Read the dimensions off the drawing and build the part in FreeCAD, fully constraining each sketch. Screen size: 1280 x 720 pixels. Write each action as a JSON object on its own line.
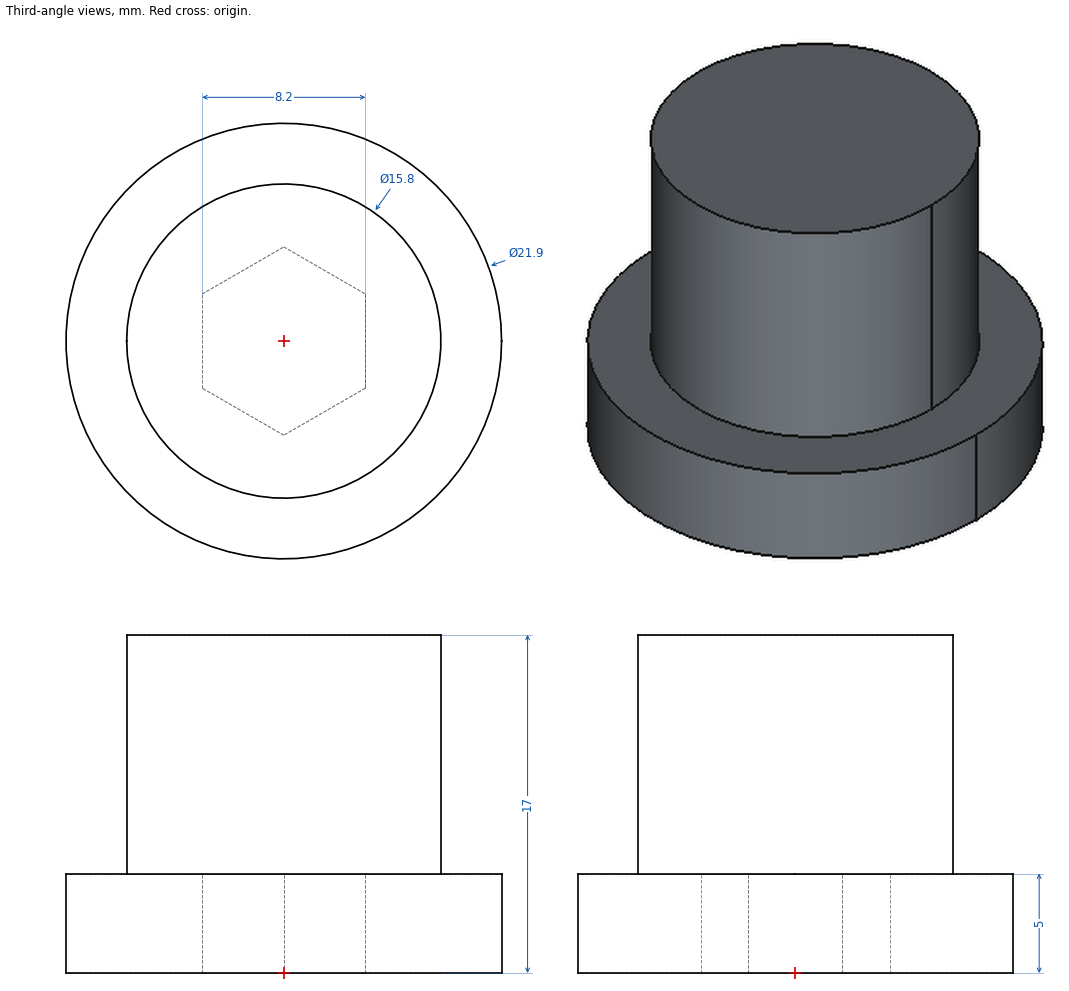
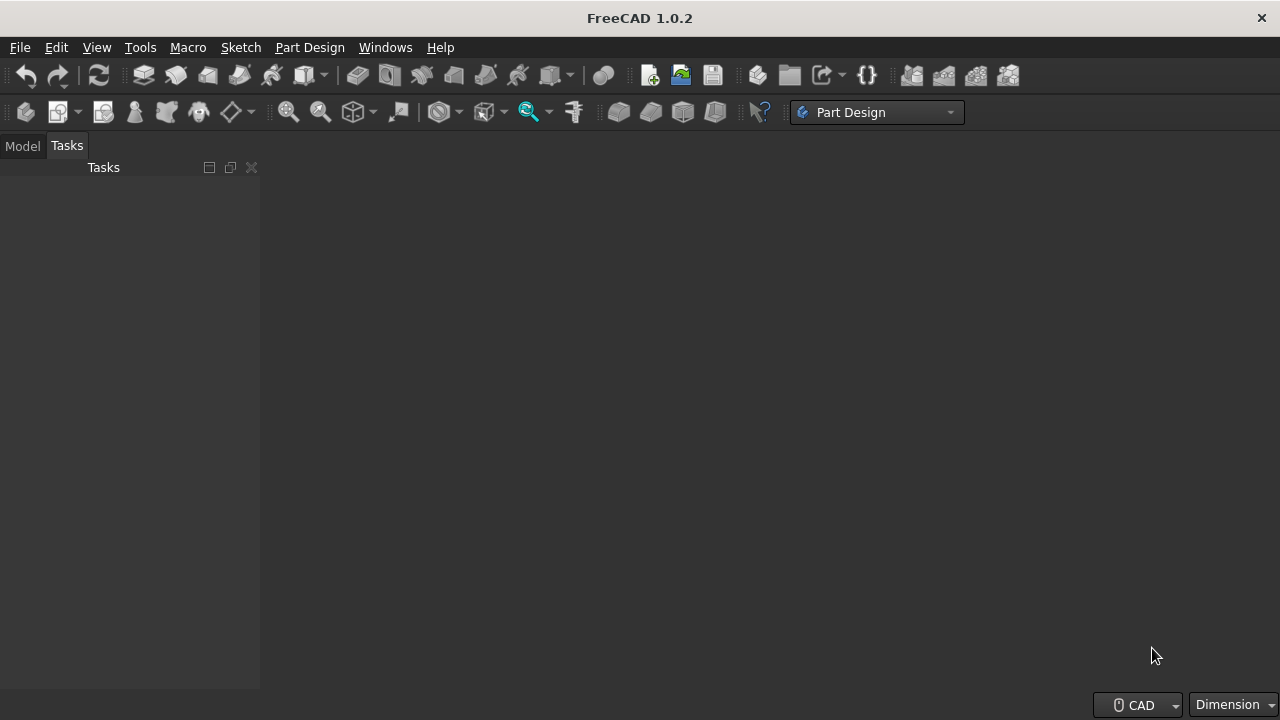
{"action": "left_click", "coordinate": [650, 76]}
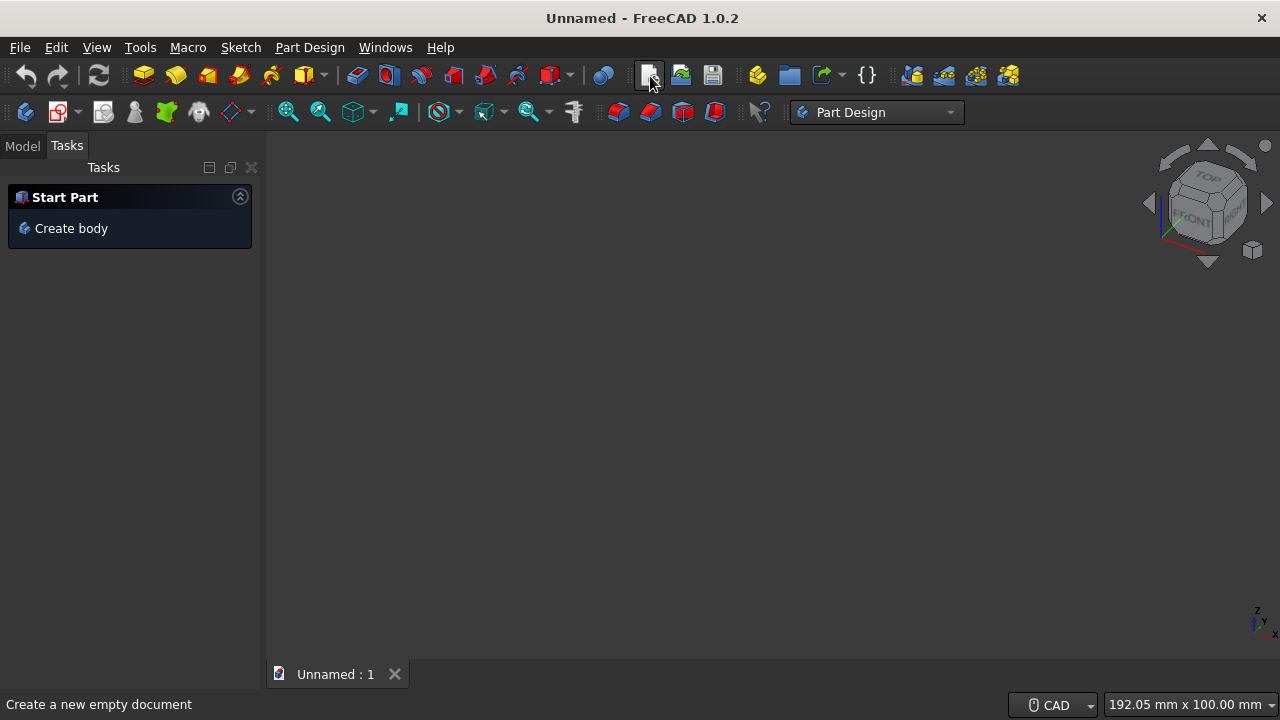
{"action": "left_click", "coordinate": [58, 112]}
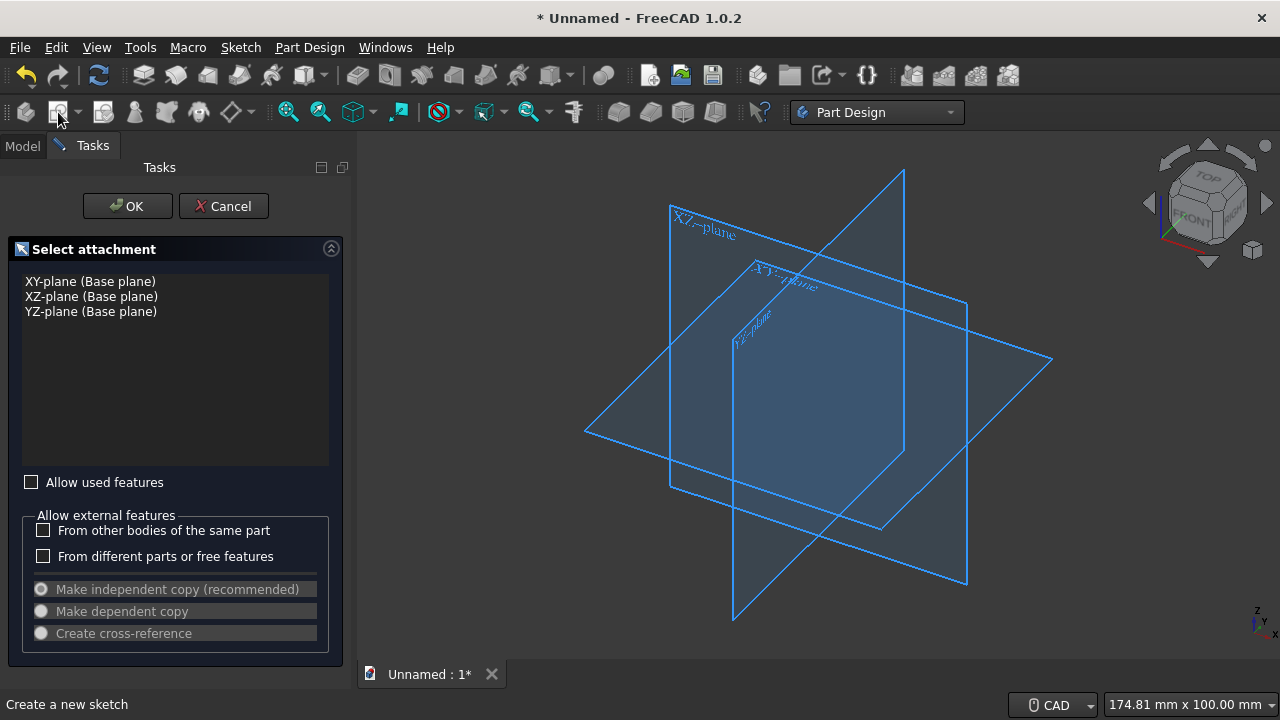
{"action": "left_click", "coordinate": [82, 282]}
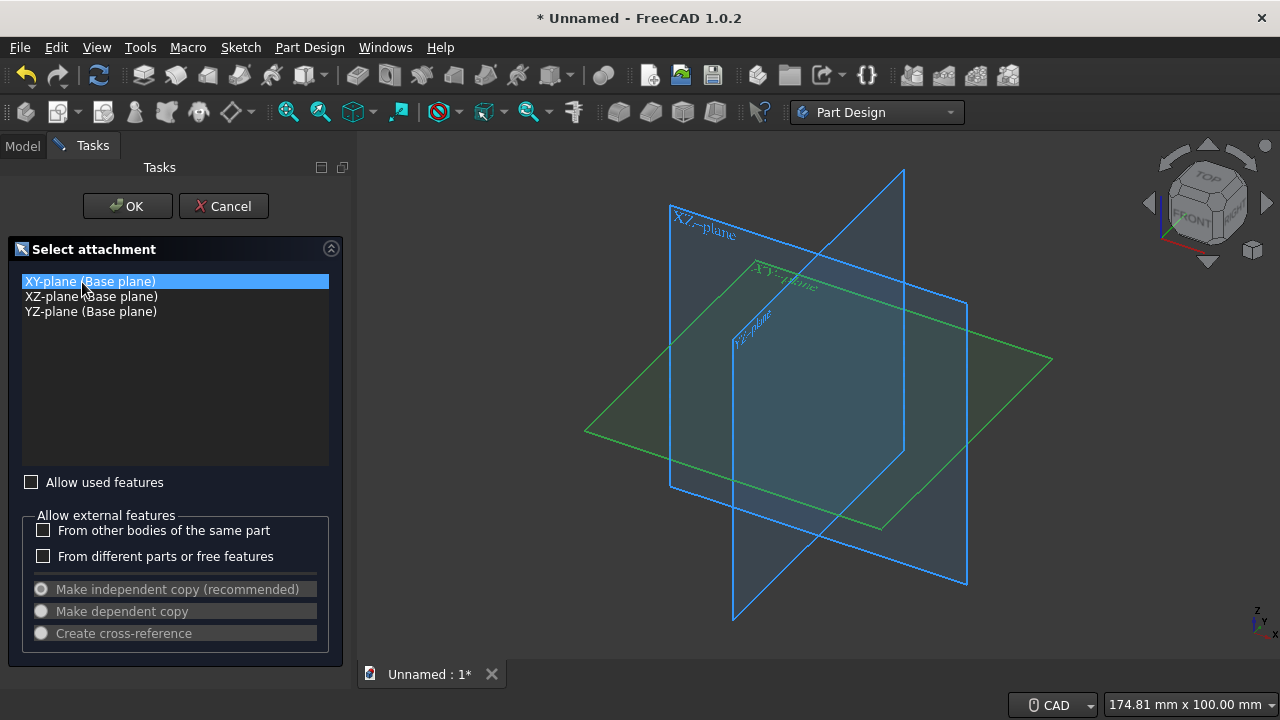
{"action": "left_click", "coordinate": [128, 206]}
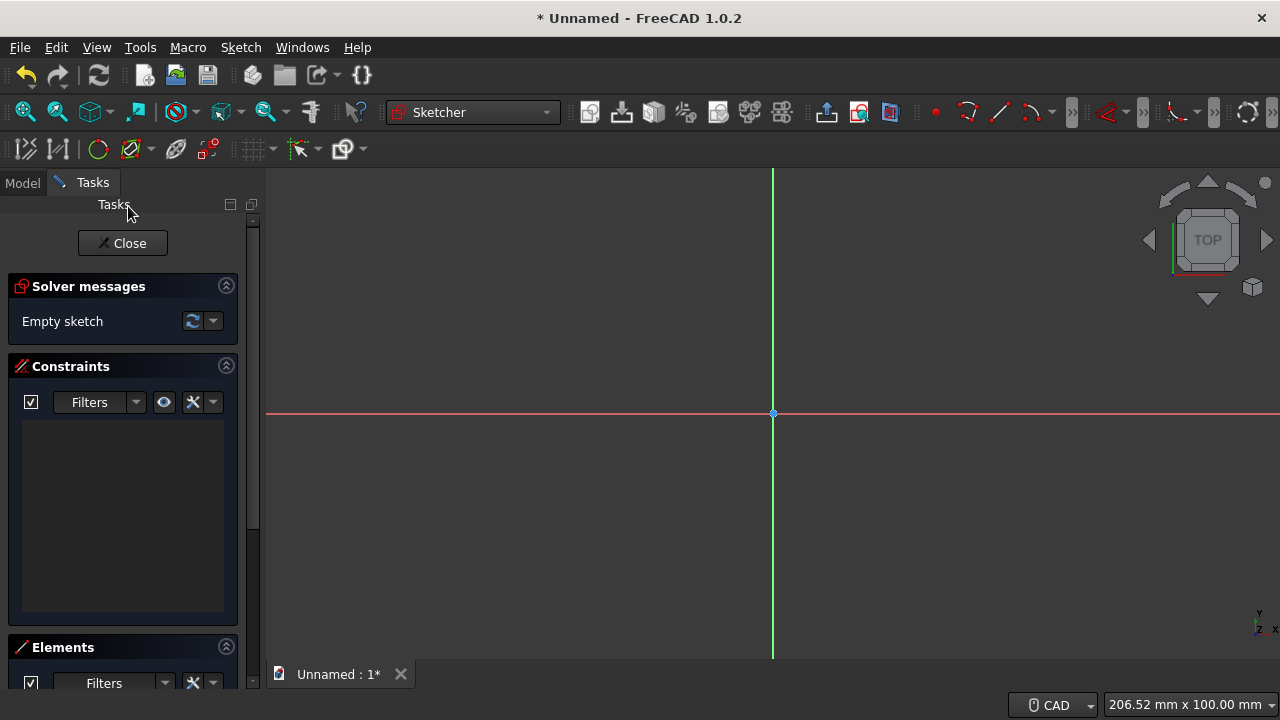
{"action": "scroll", "coordinate": [813, 414], "scroll_direction": "up", "scroll_amount": 5}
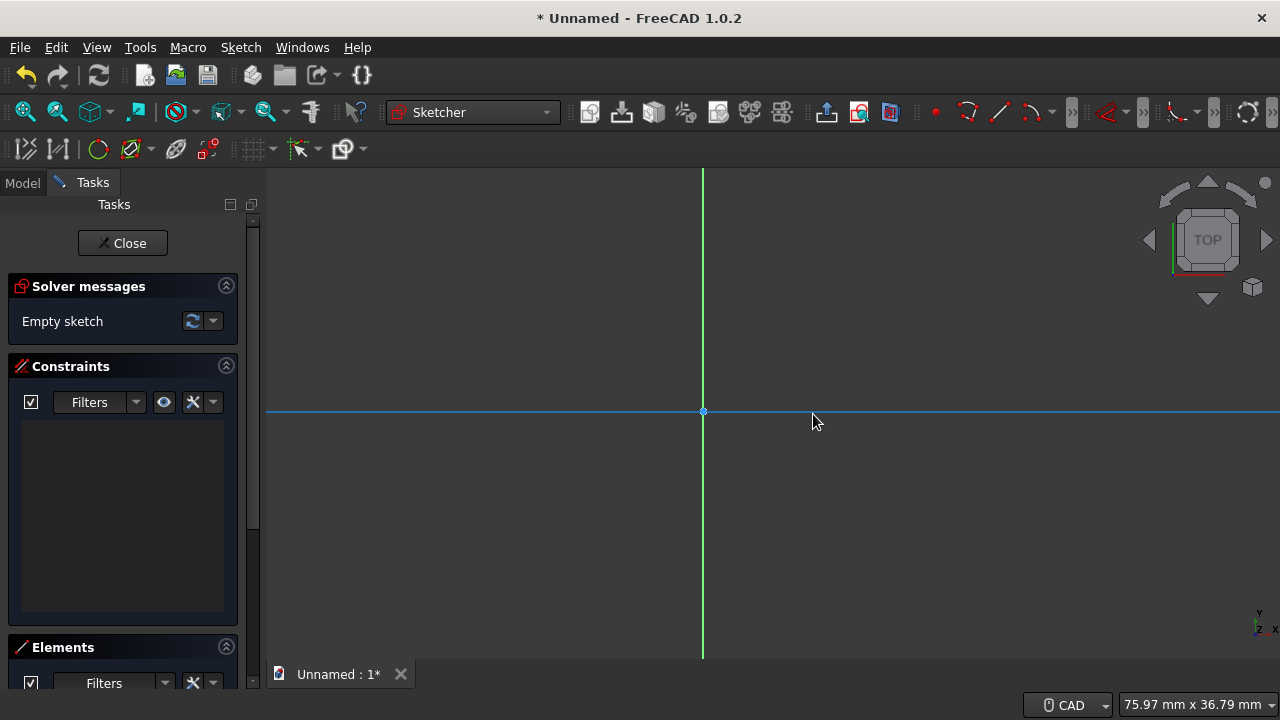
{"action": "key", "text": "g c"}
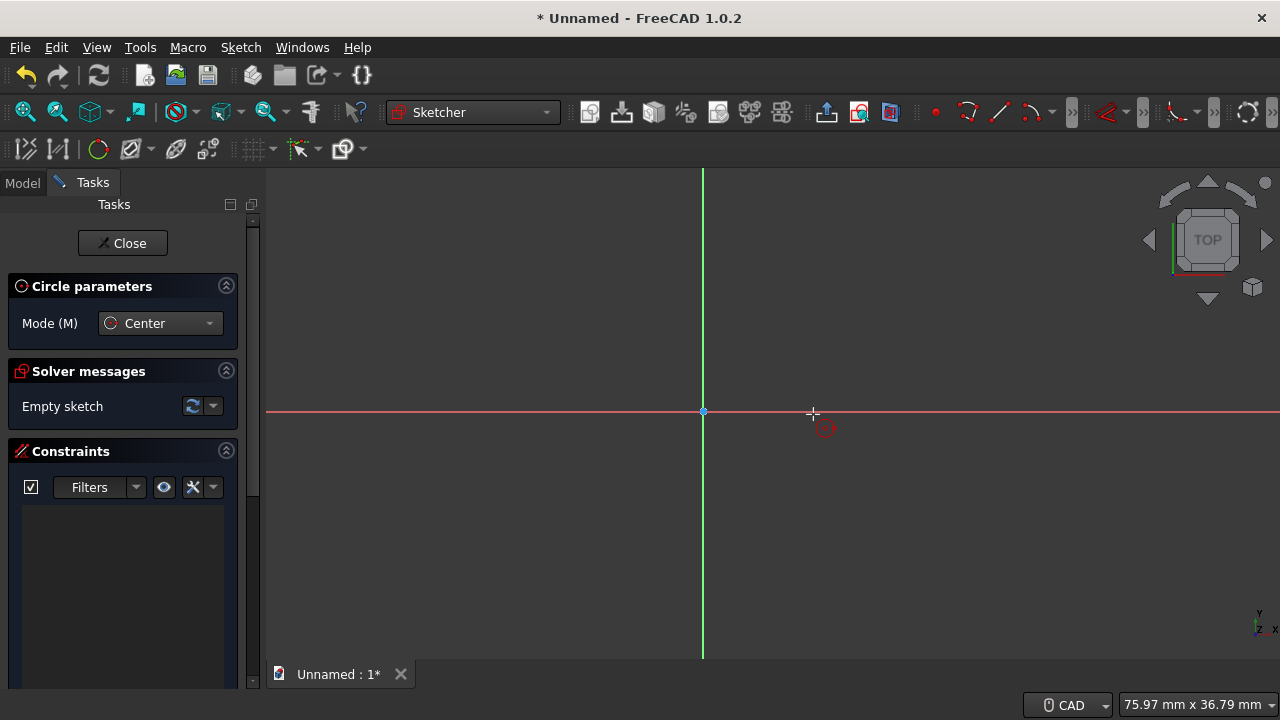
{"action": "left_click", "coordinate": [703, 412]}
{"action": "mouse_move", "coordinate": [807, 308]}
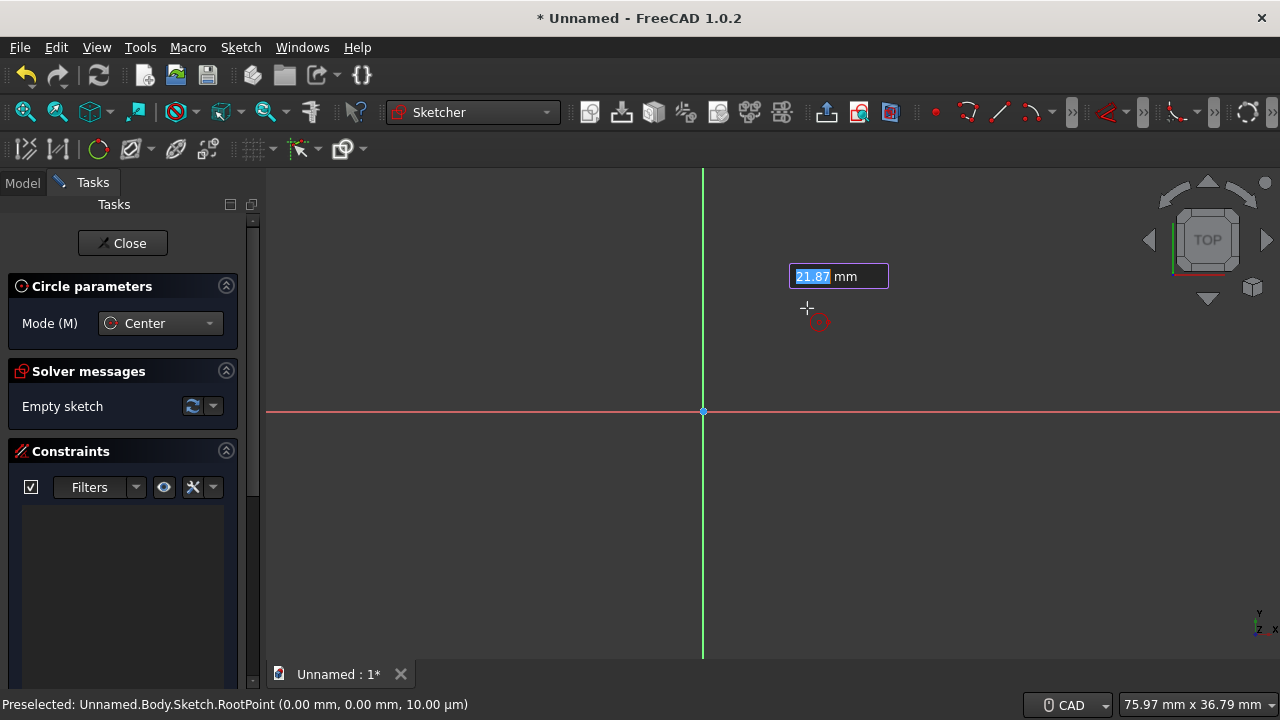
{"action": "type", "text": "21.9"}
{"action": "key", "text": "Return"}
{"action": "key", "text": "Escape"}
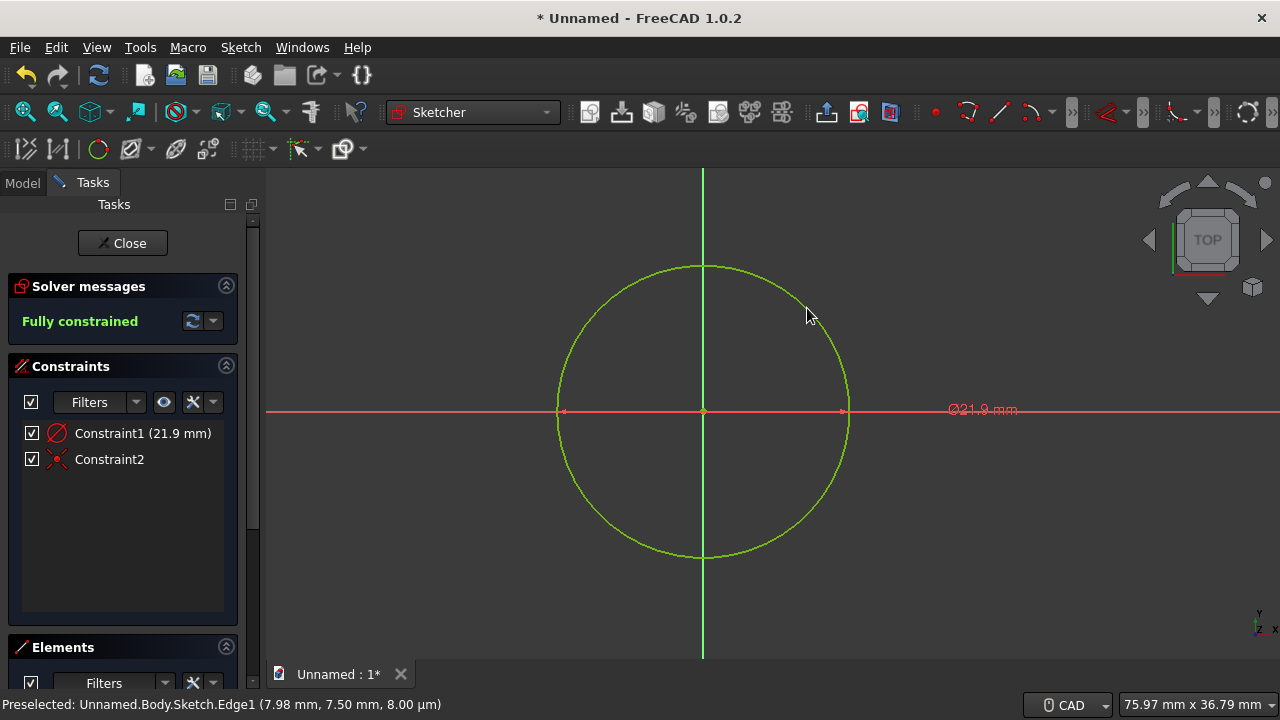
{"action": "left_click", "coordinate": [123, 243]}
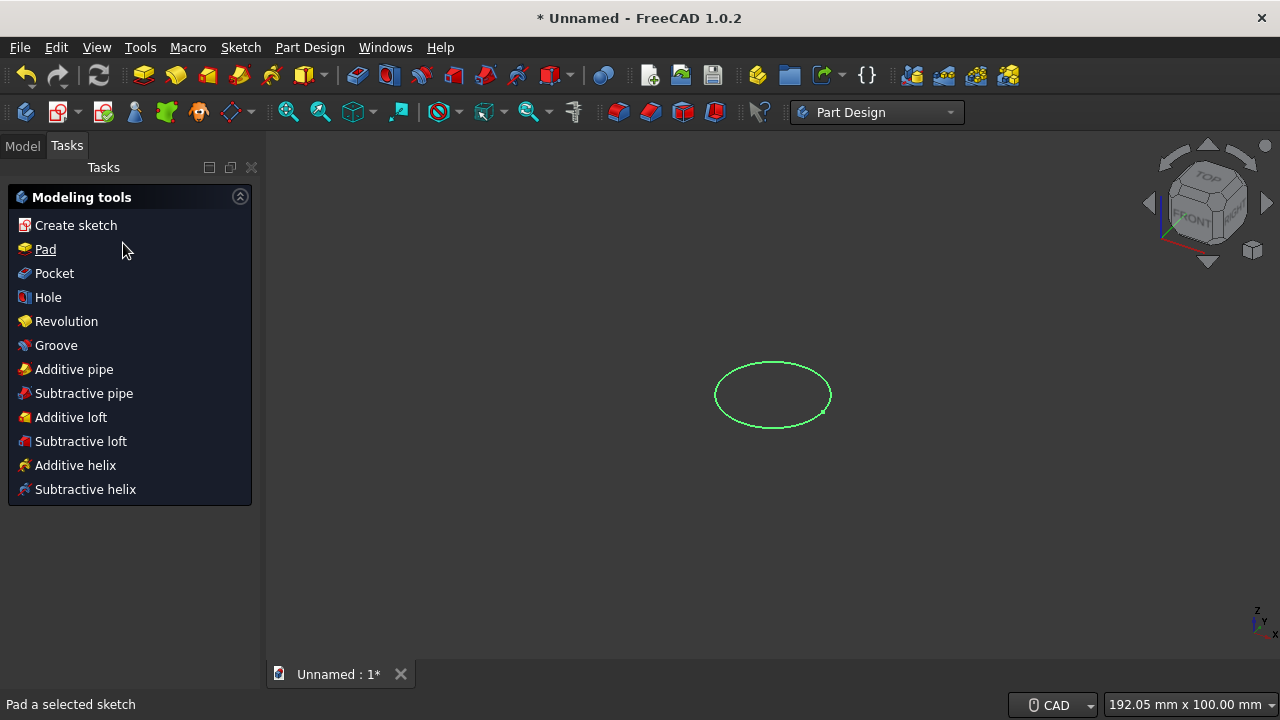
{"action": "left_click", "coordinate": [144, 76]}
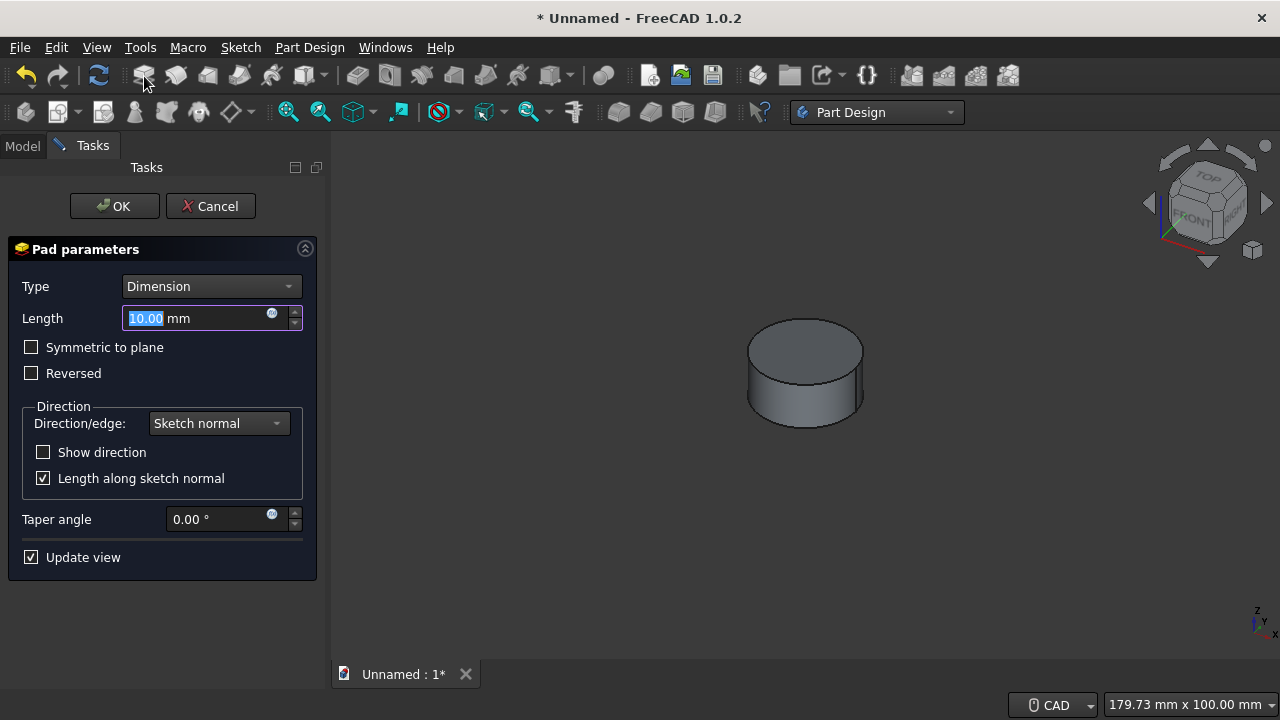
{"action": "type", "text": "5"}
{"action": "key", "text": "Tab"}